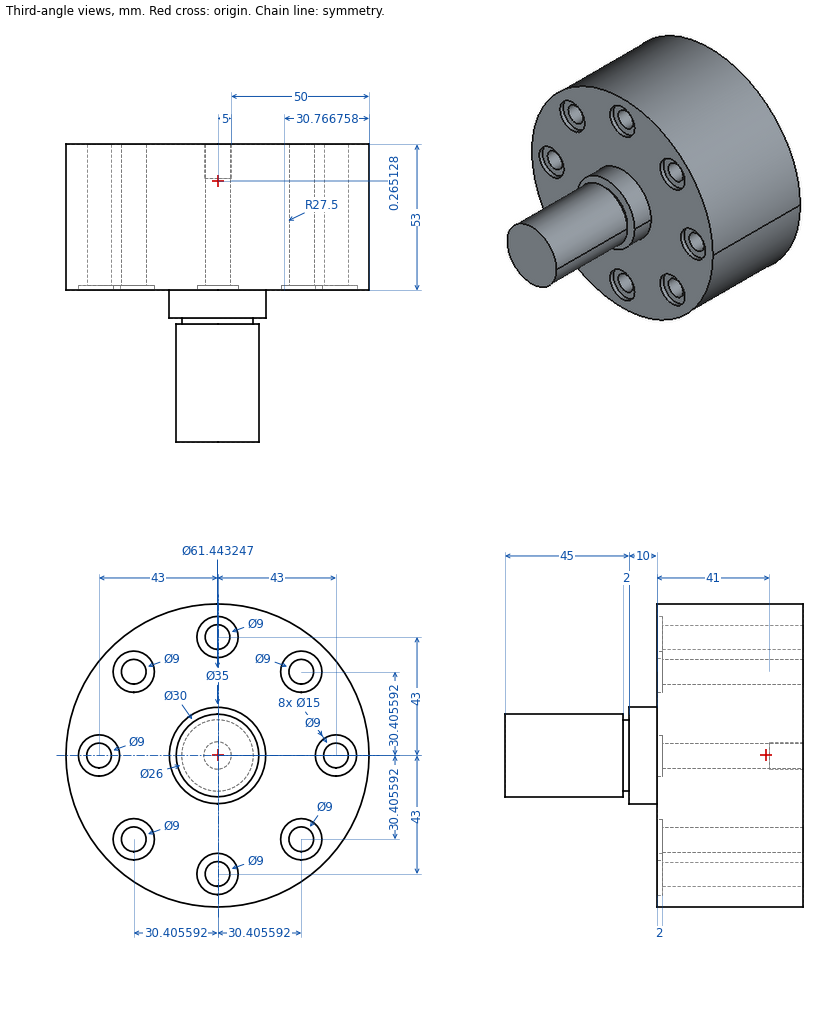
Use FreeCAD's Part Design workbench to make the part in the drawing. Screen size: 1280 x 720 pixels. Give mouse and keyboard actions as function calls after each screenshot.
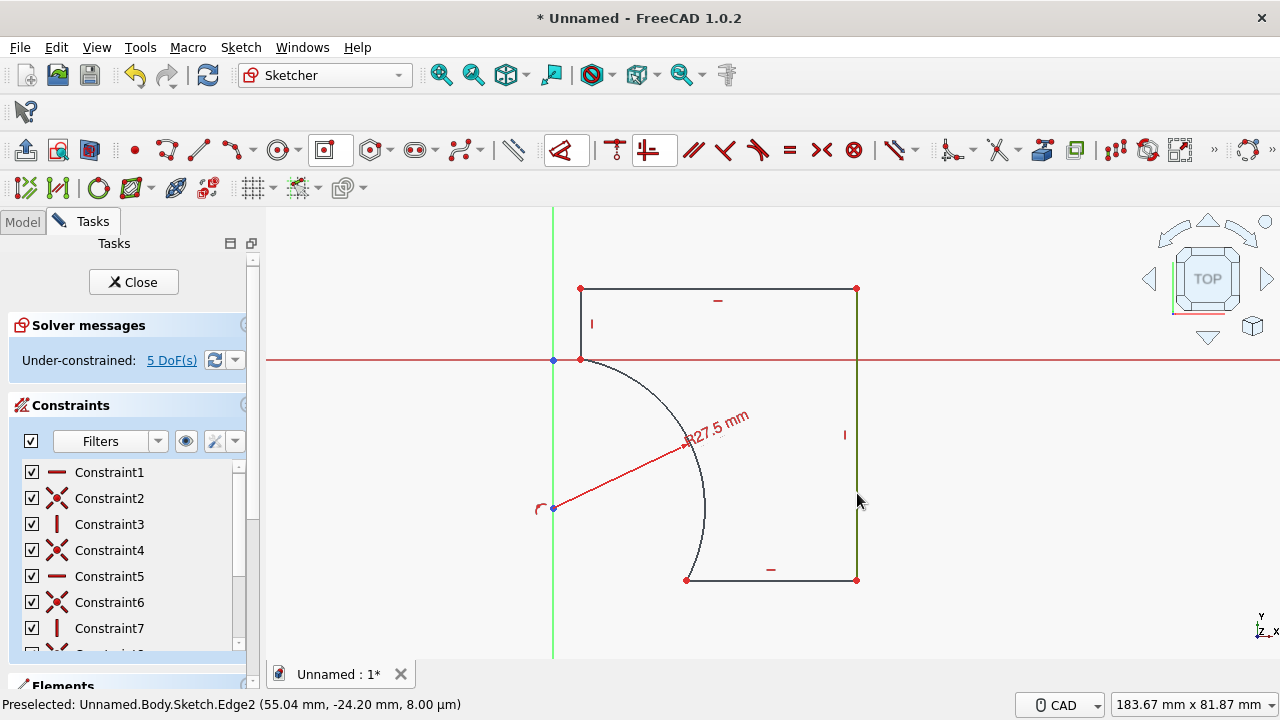
key(i)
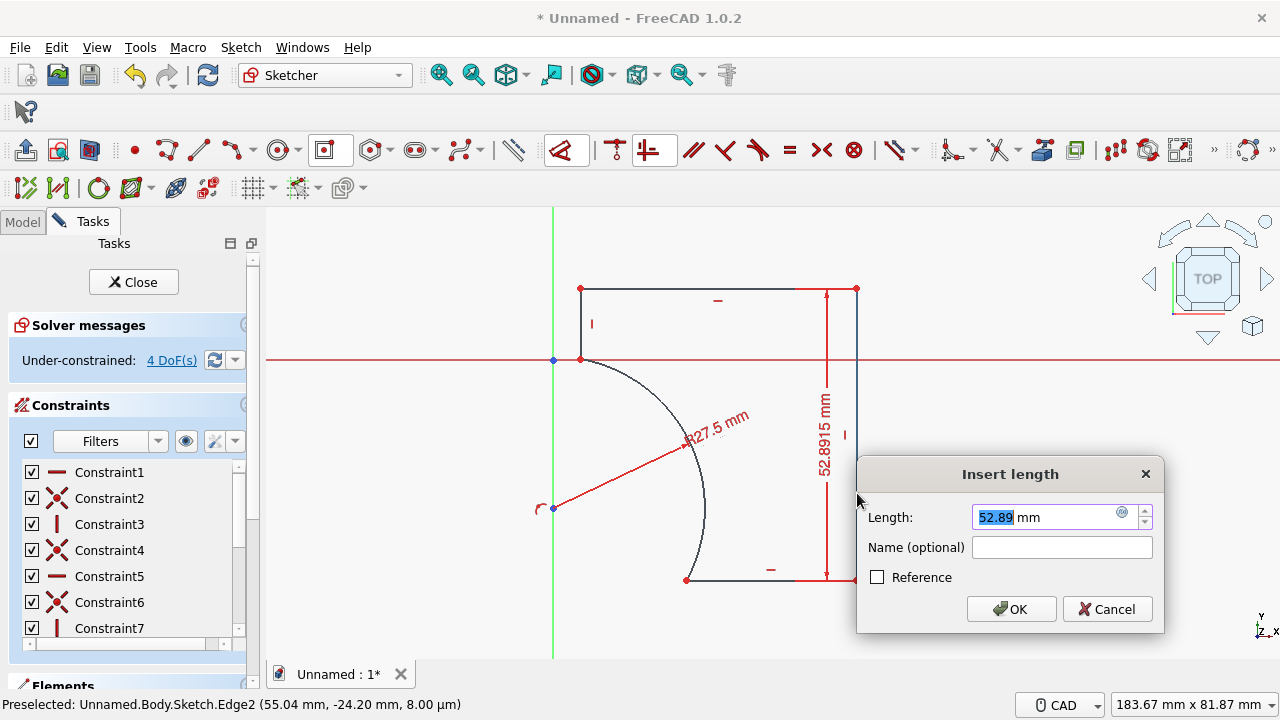
text(53)
key(Return)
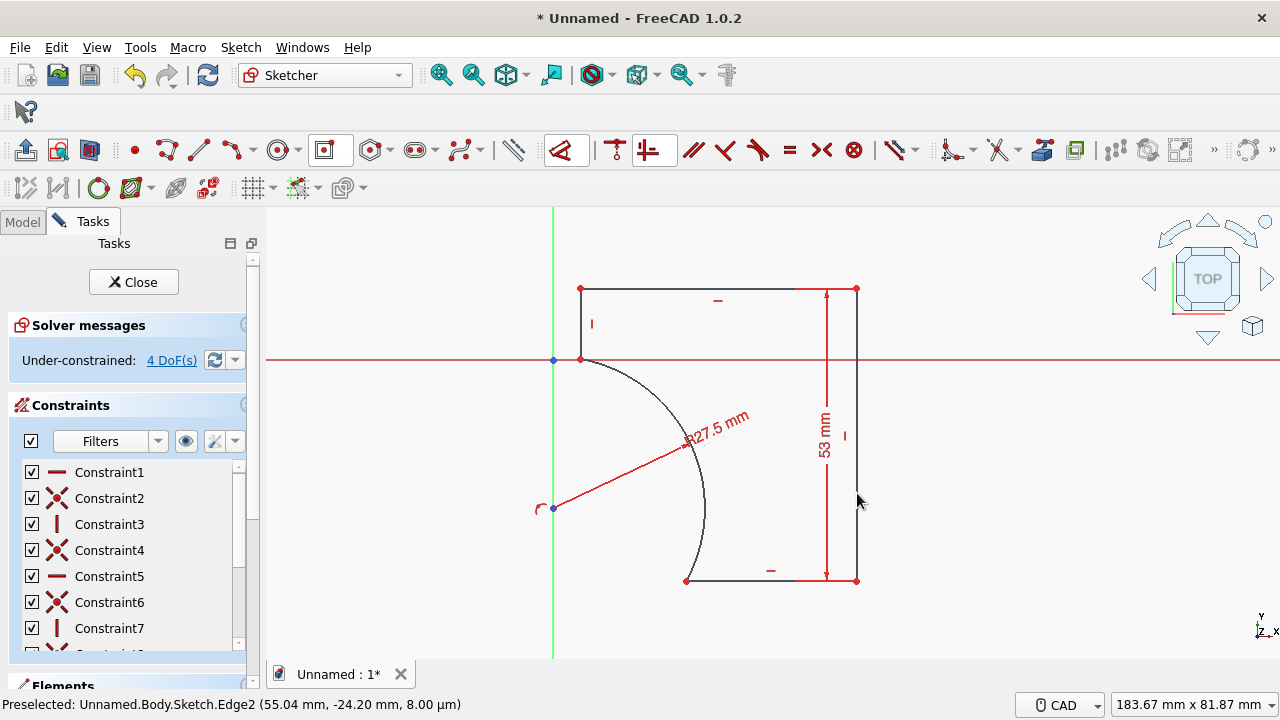
click(774, 289)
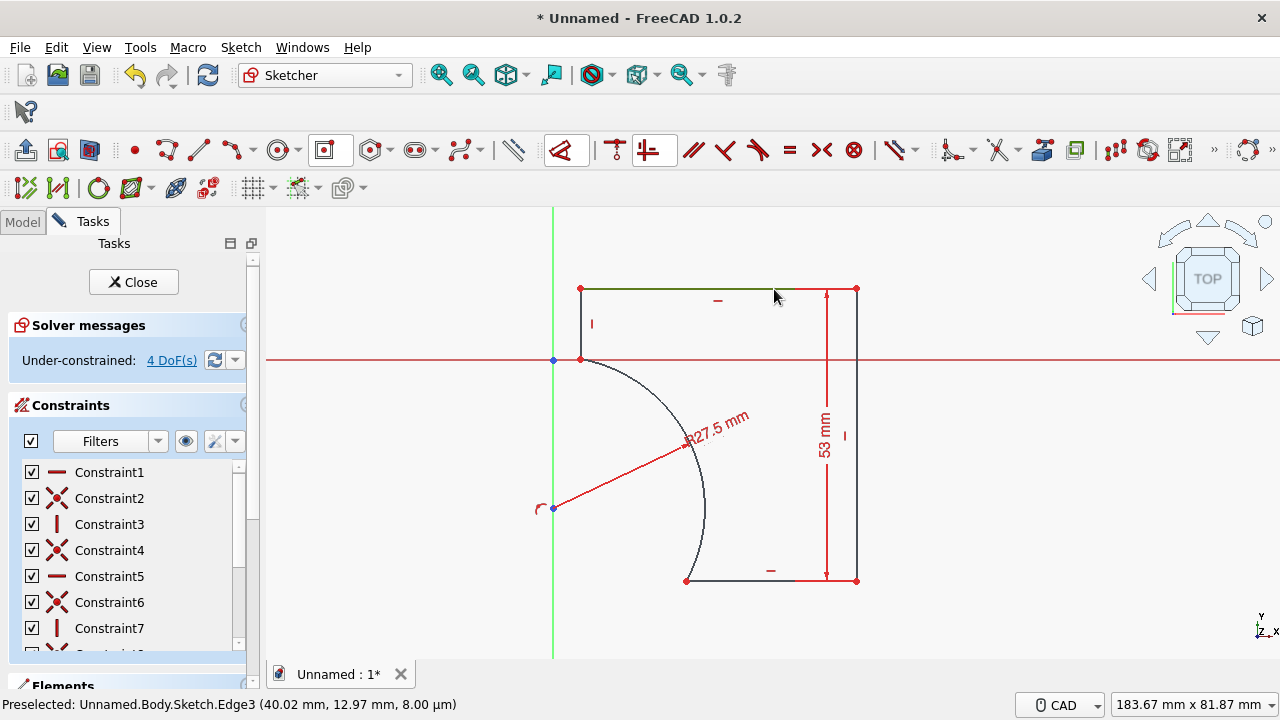
key(l)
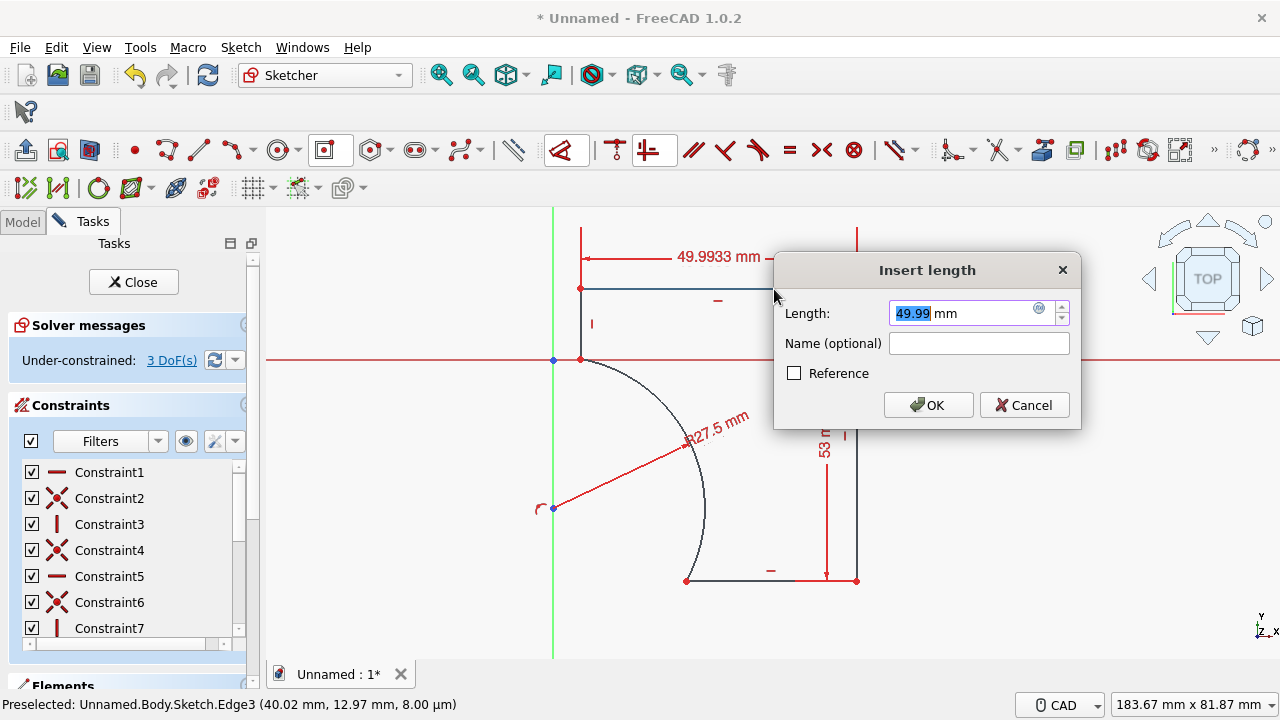
text(50)
key(Return)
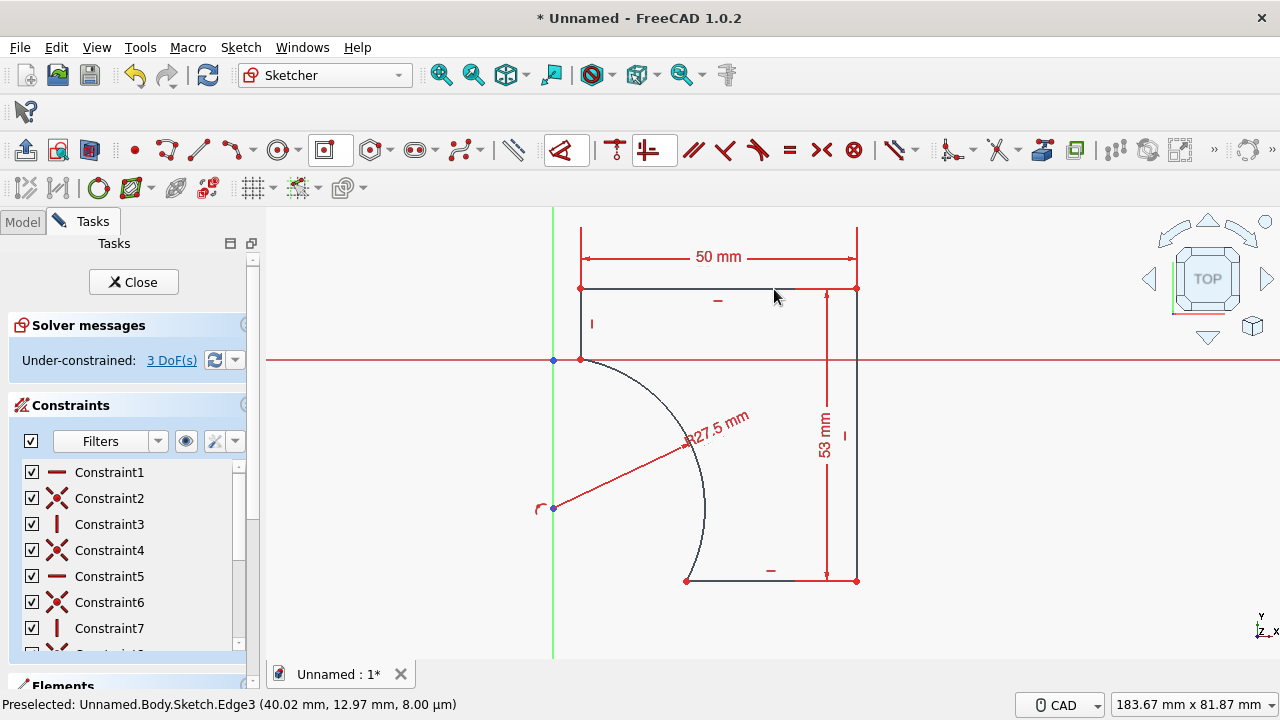
scroll(581, 289, up, 2)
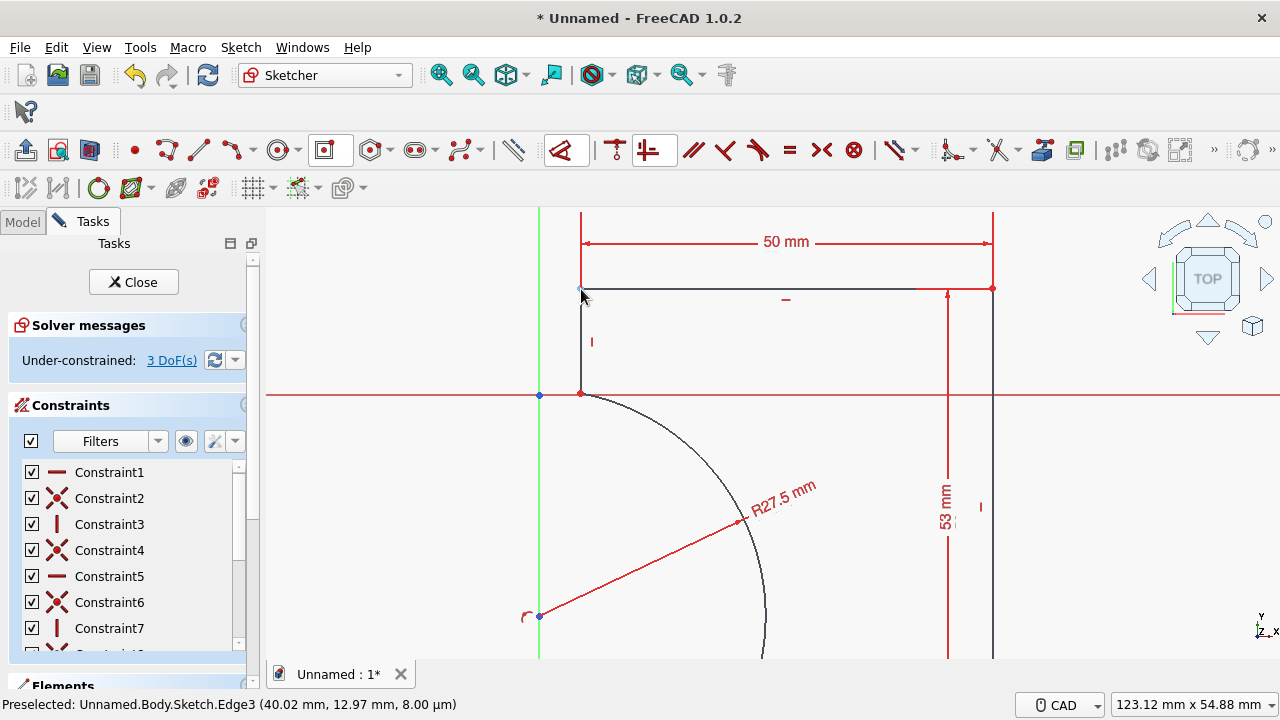
click(581, 289)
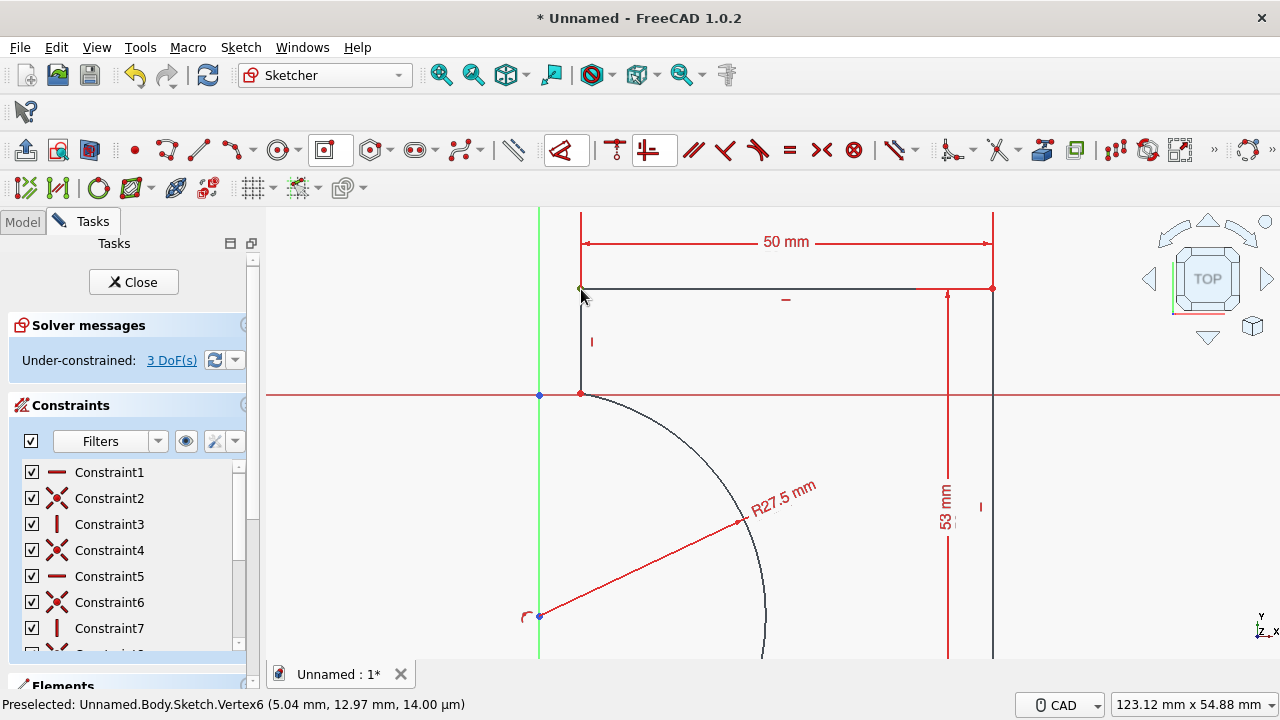
click(584, 150)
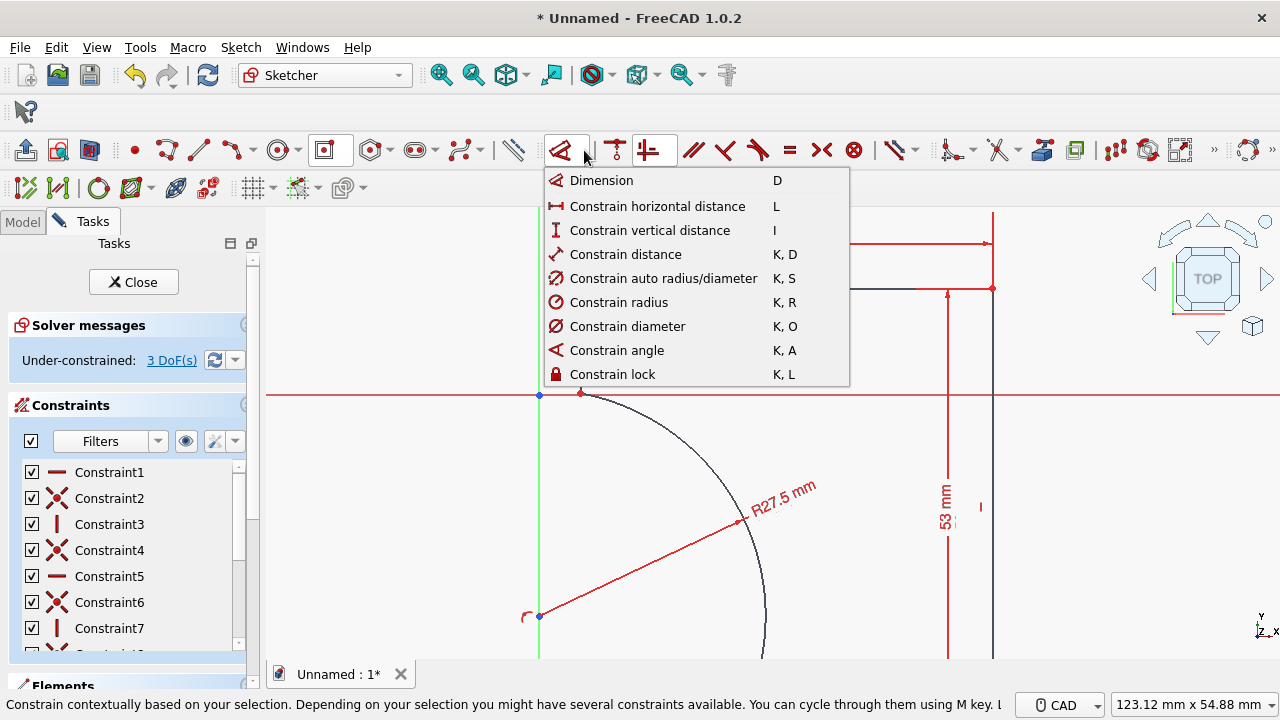
click(697, 206)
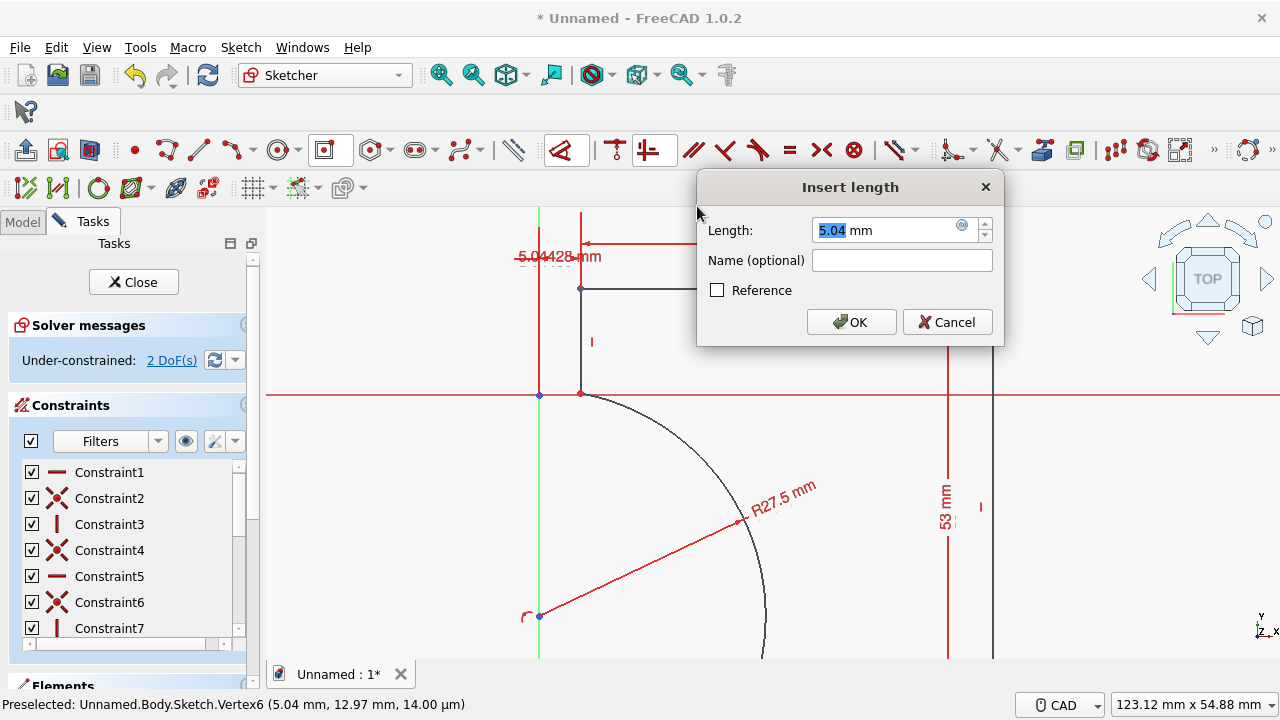
text(5)
key(Return)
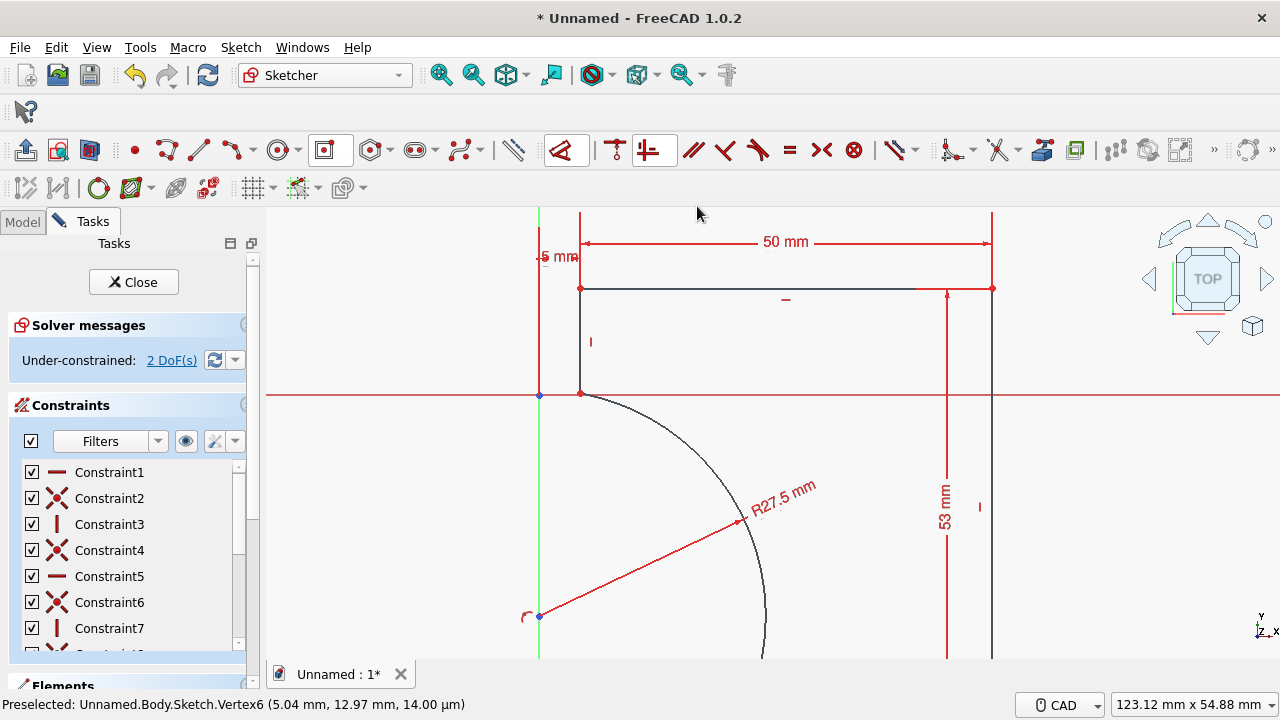
scroll(580, 287, down, 2)